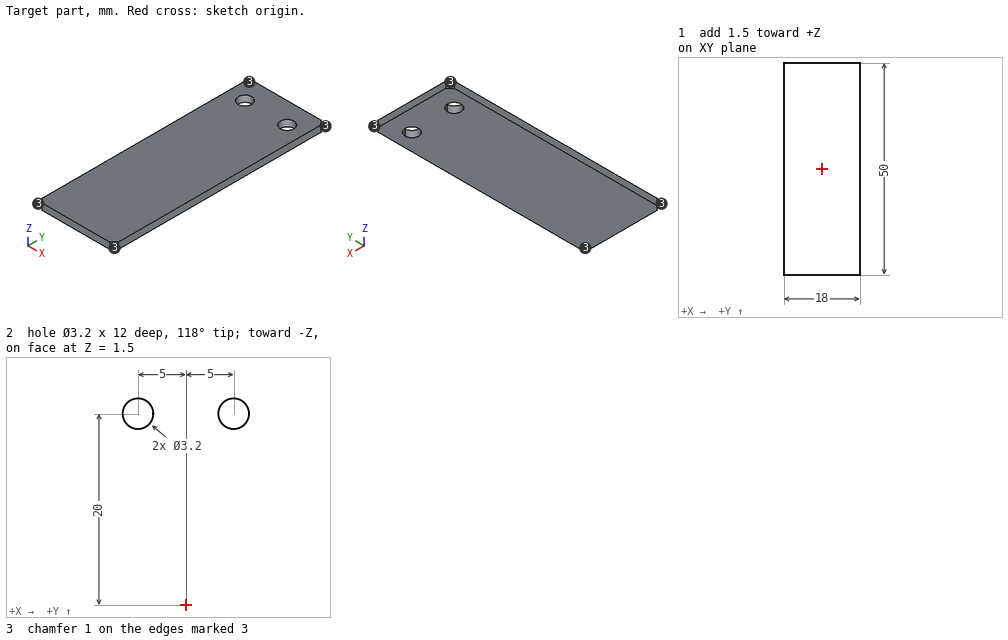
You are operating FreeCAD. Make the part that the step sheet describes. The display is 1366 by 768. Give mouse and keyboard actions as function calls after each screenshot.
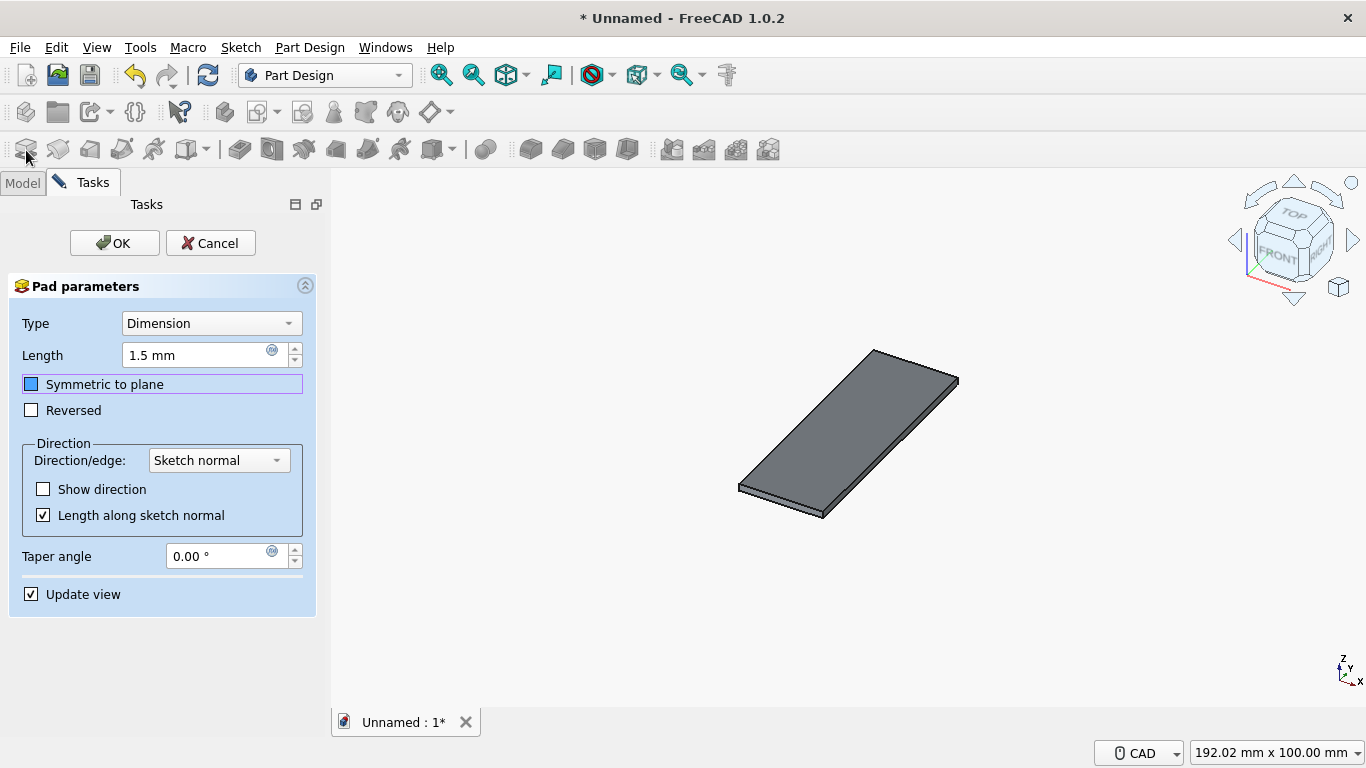
click(115, 243)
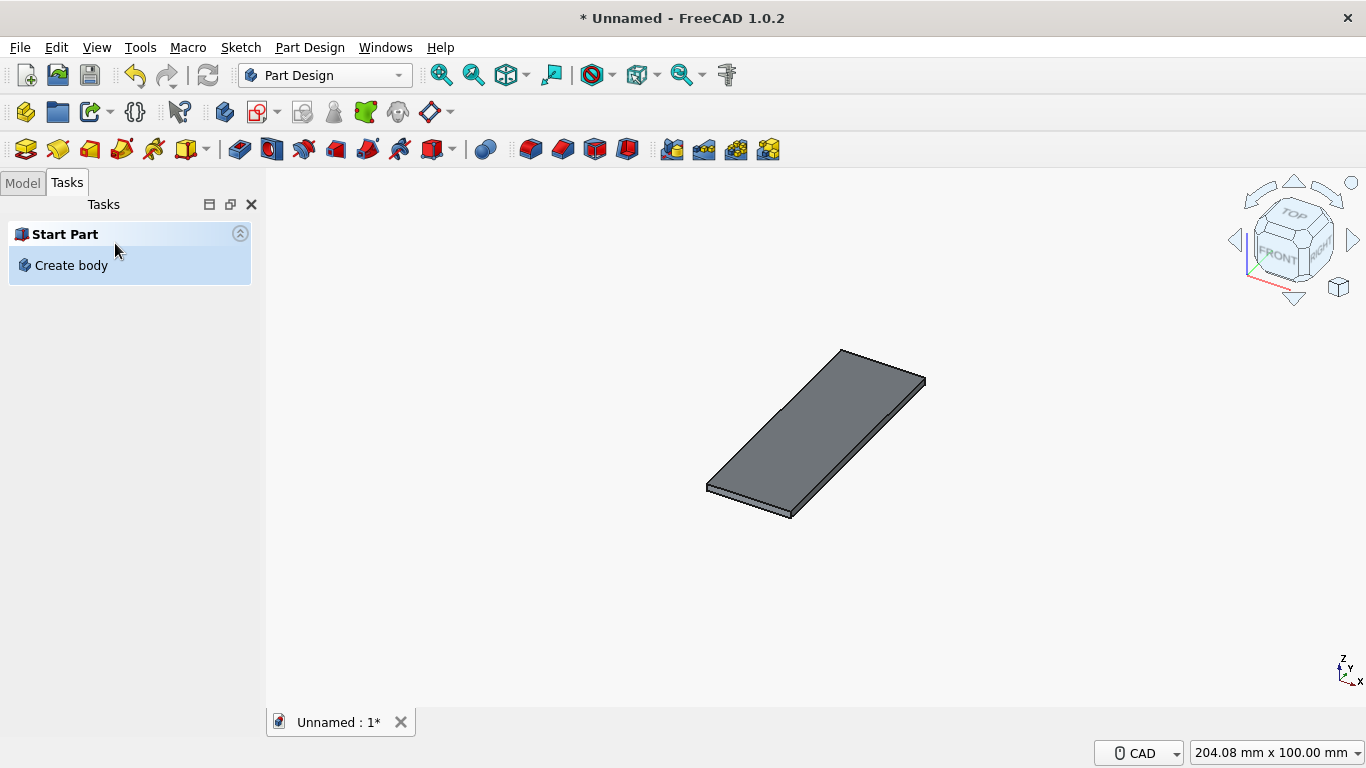
click(442, 76)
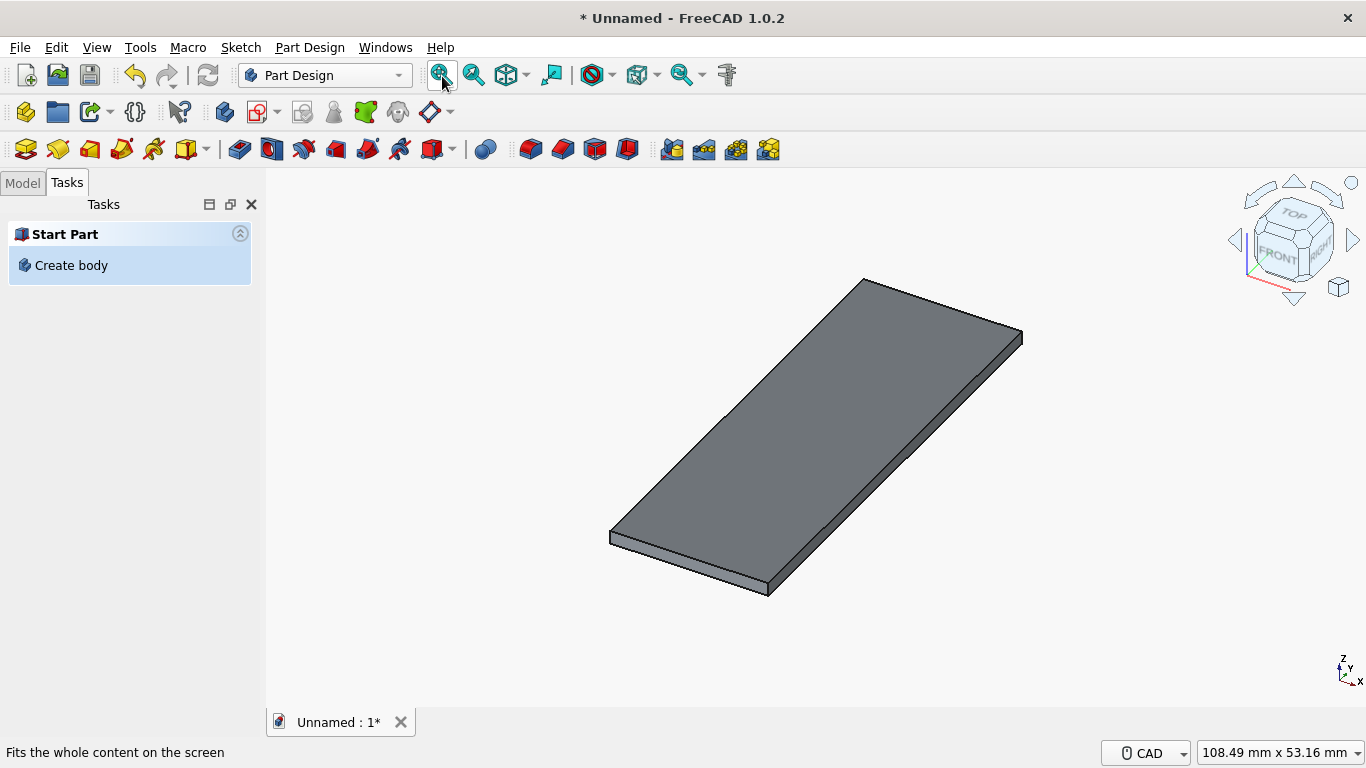
click(888, 358)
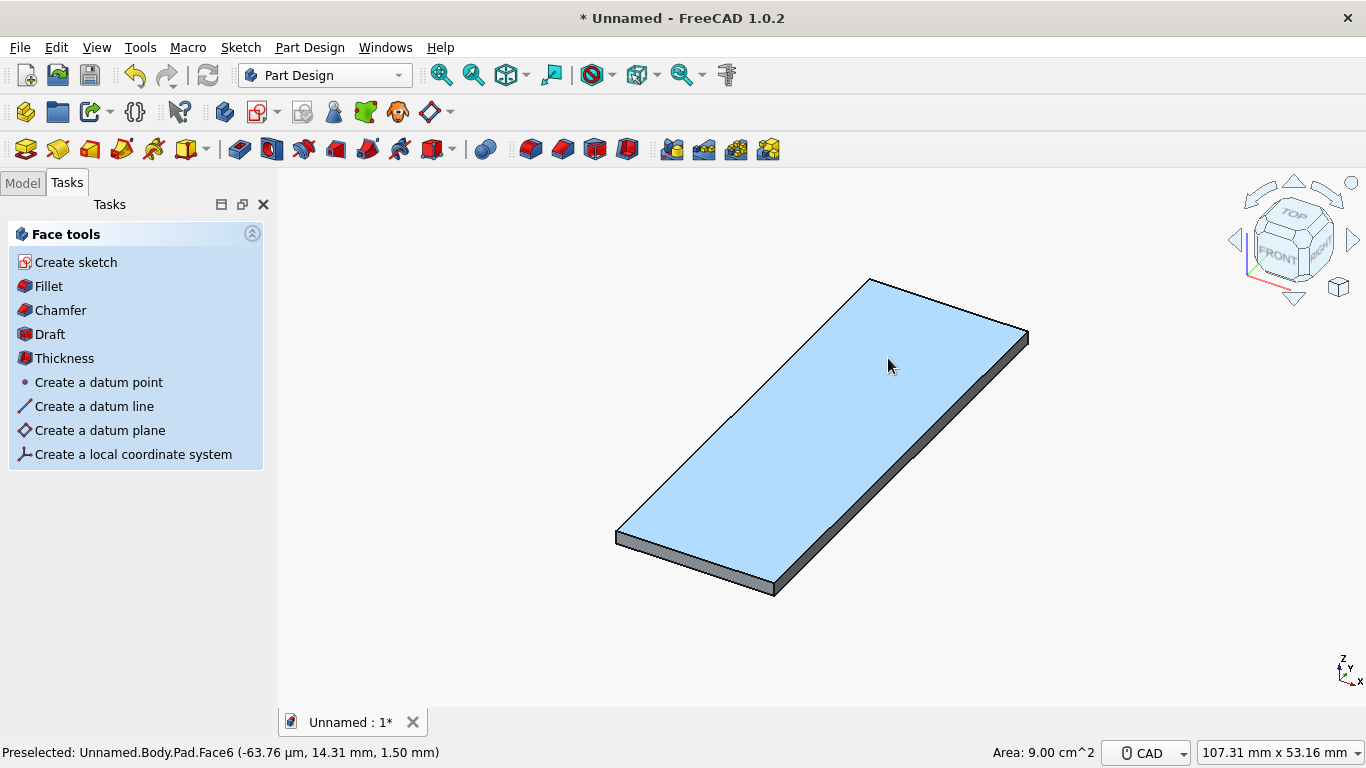
click(258, 112)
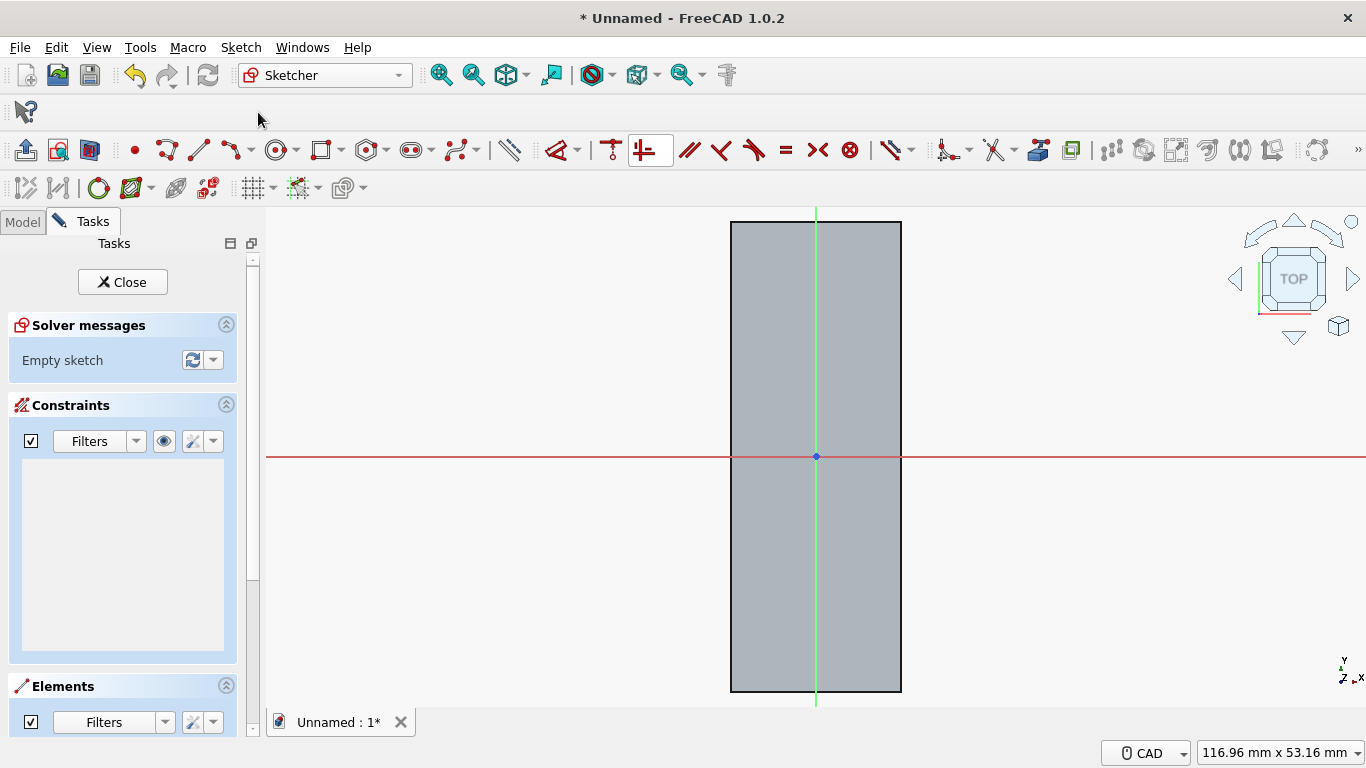
scroll(955, 235, up, 2)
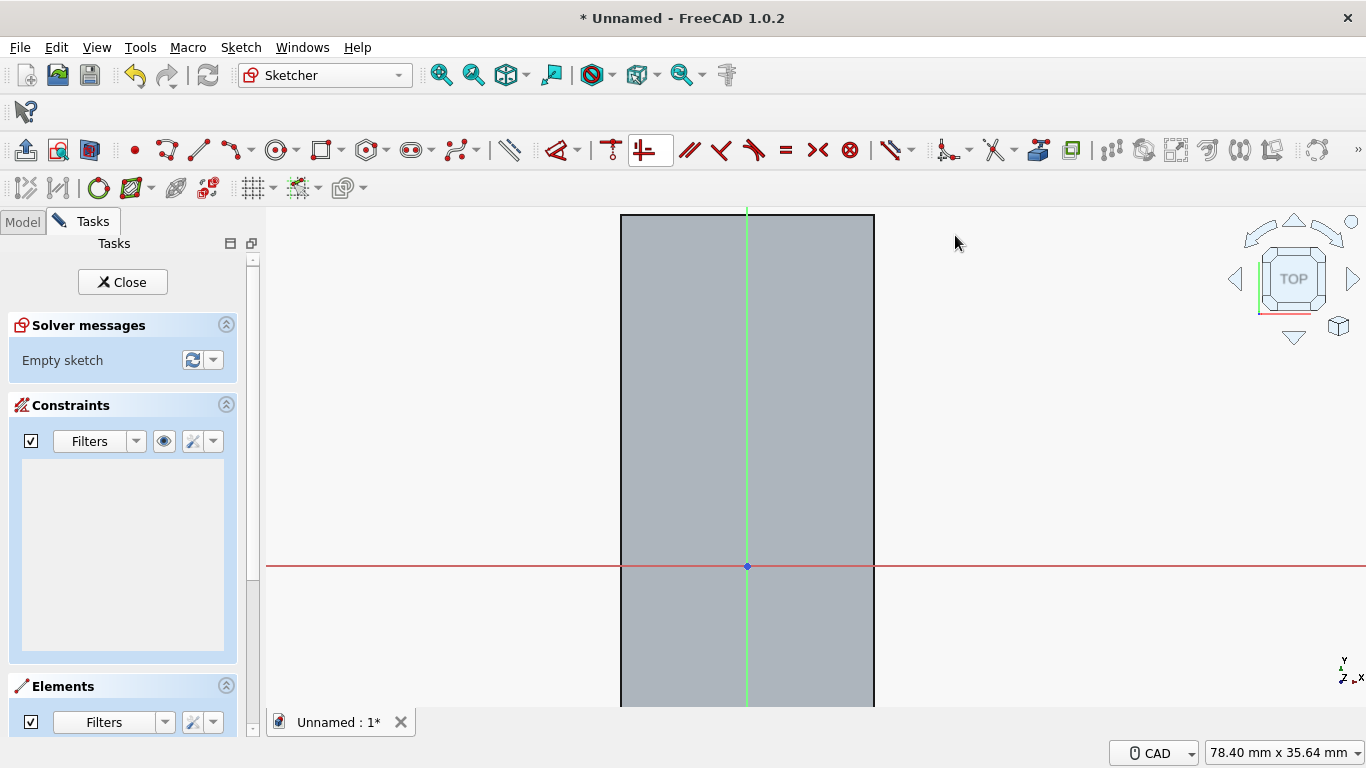
click(276, 150)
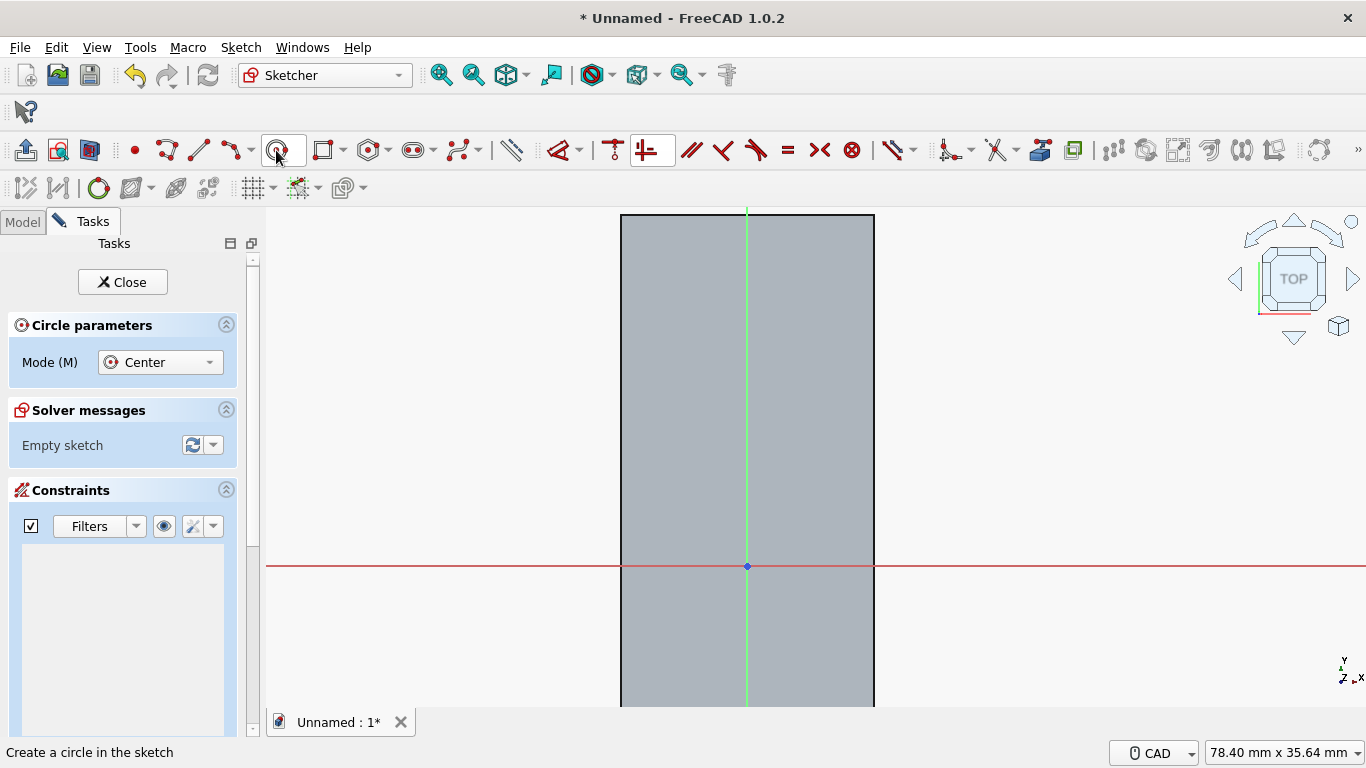
click(677, 286)
move(693, 270)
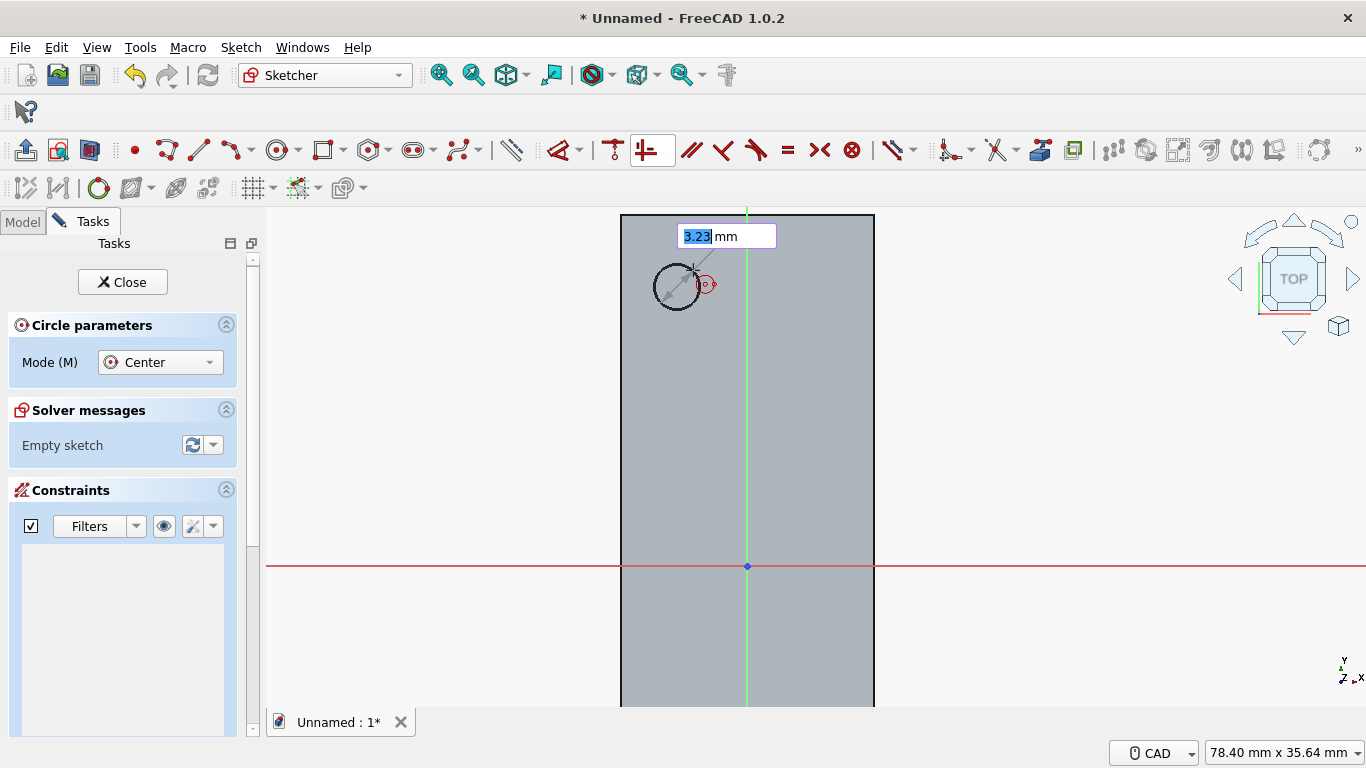
text(3.2)
key(Return)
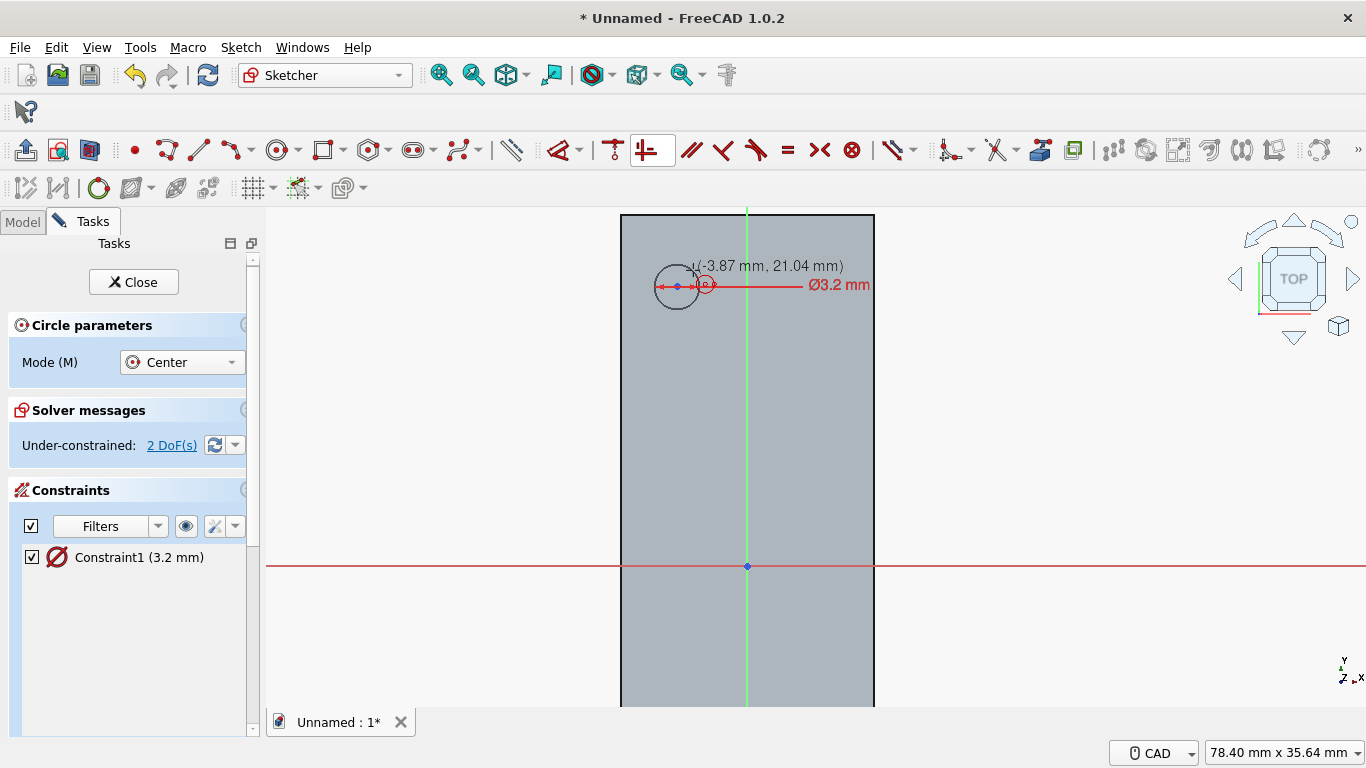
click(817, 286)
move(833, 270)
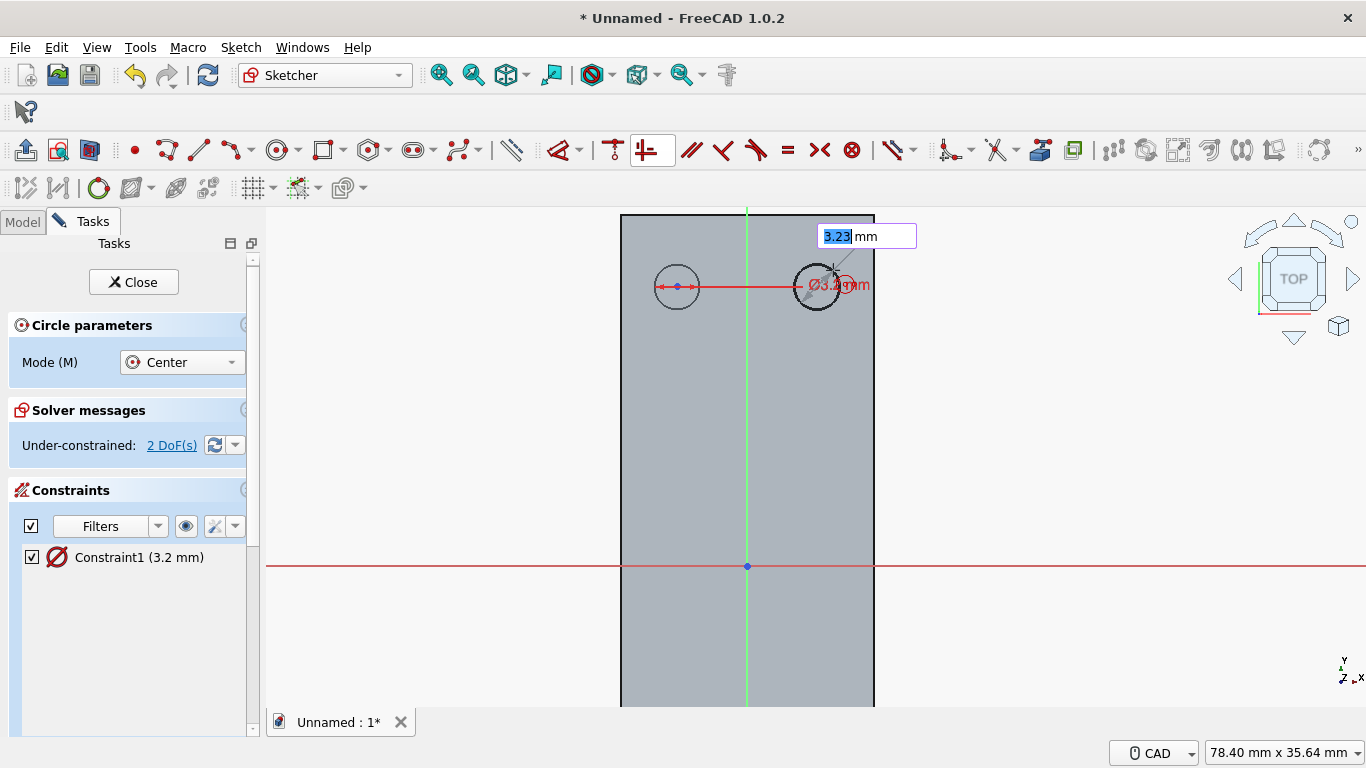
text(3.2)
key(Return)
key(Escape)